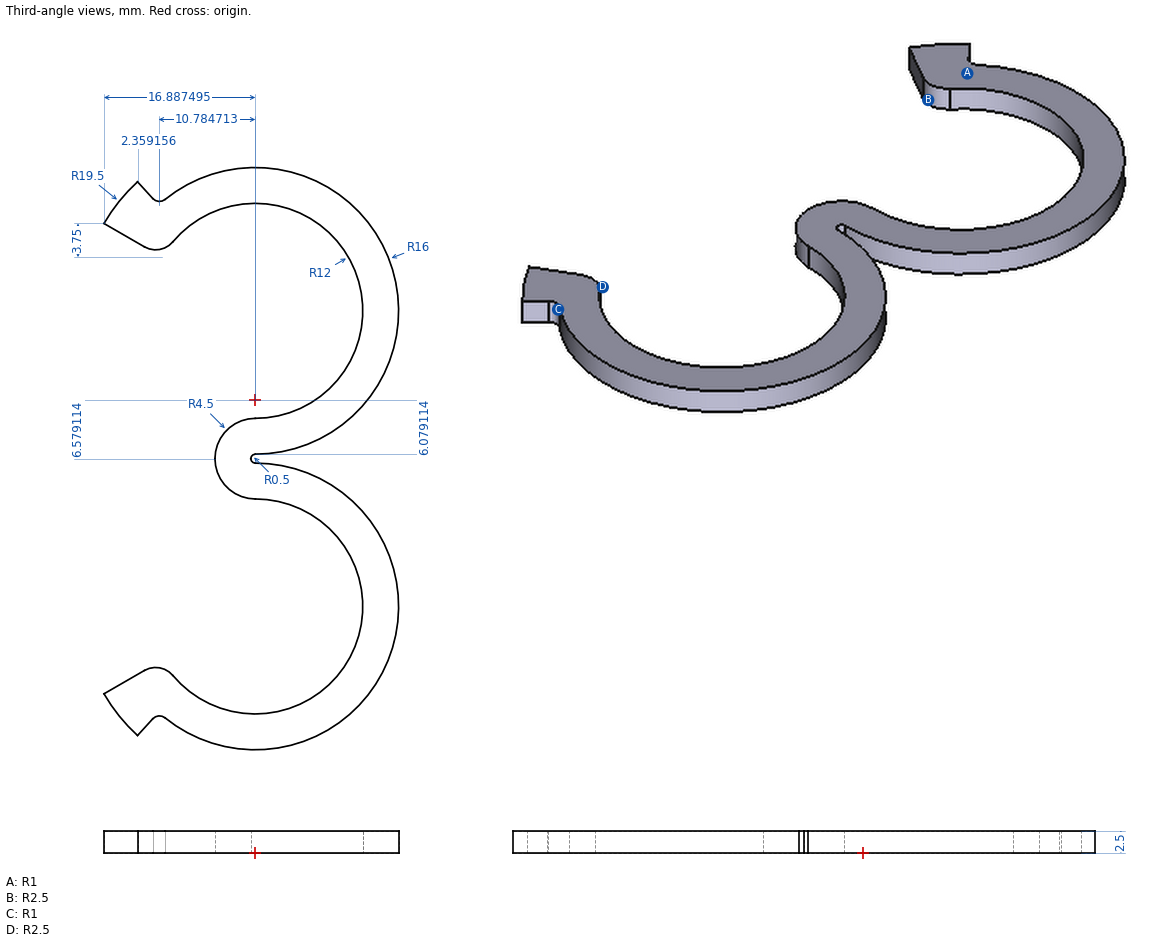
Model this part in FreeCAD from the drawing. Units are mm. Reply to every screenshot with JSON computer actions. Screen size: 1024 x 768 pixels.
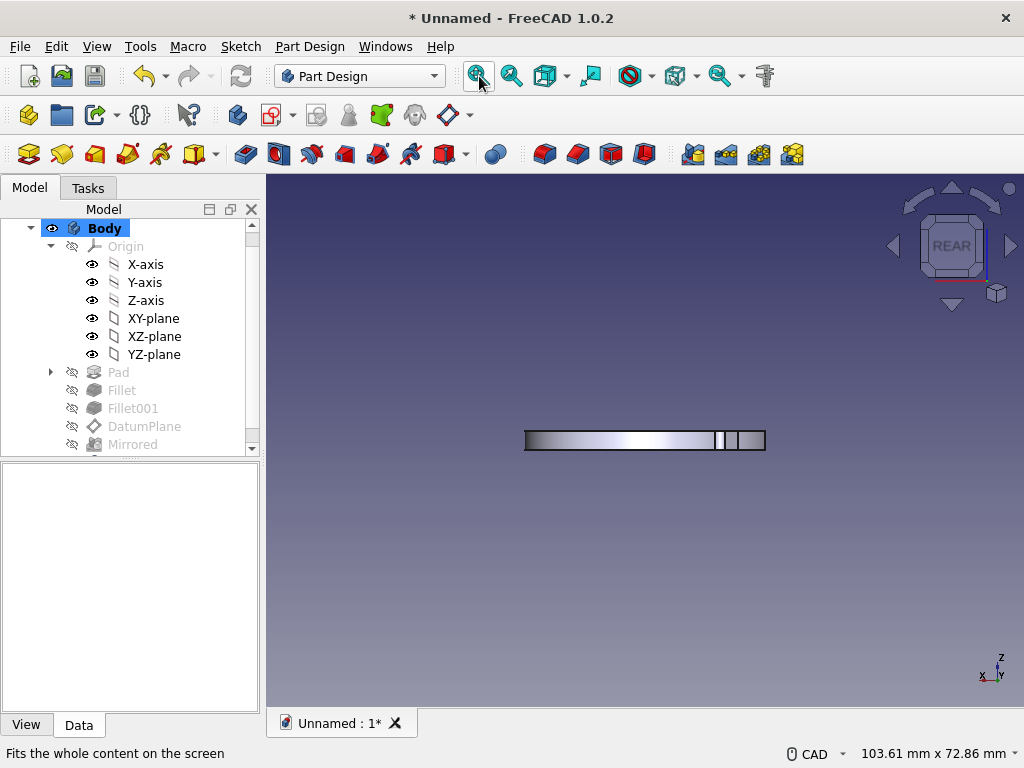
{"action": "key", "text": "6"}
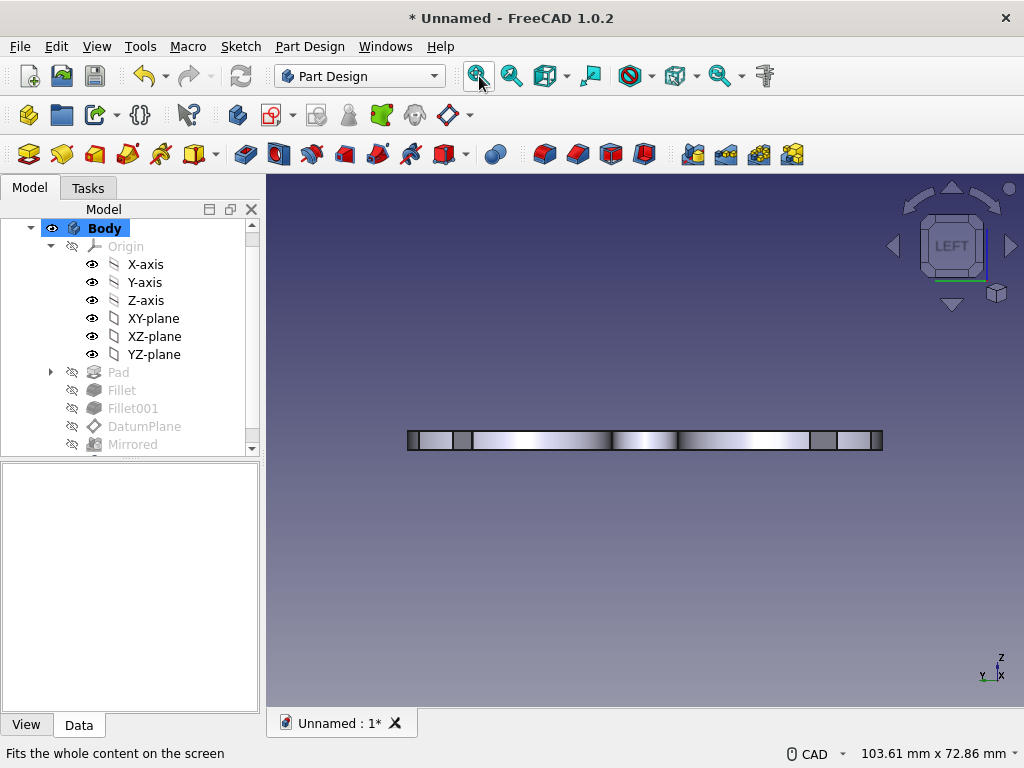
{"action": "scroll", "coordinate": [810, 439], "scroll_direction": "up", "scroll_amount": 4}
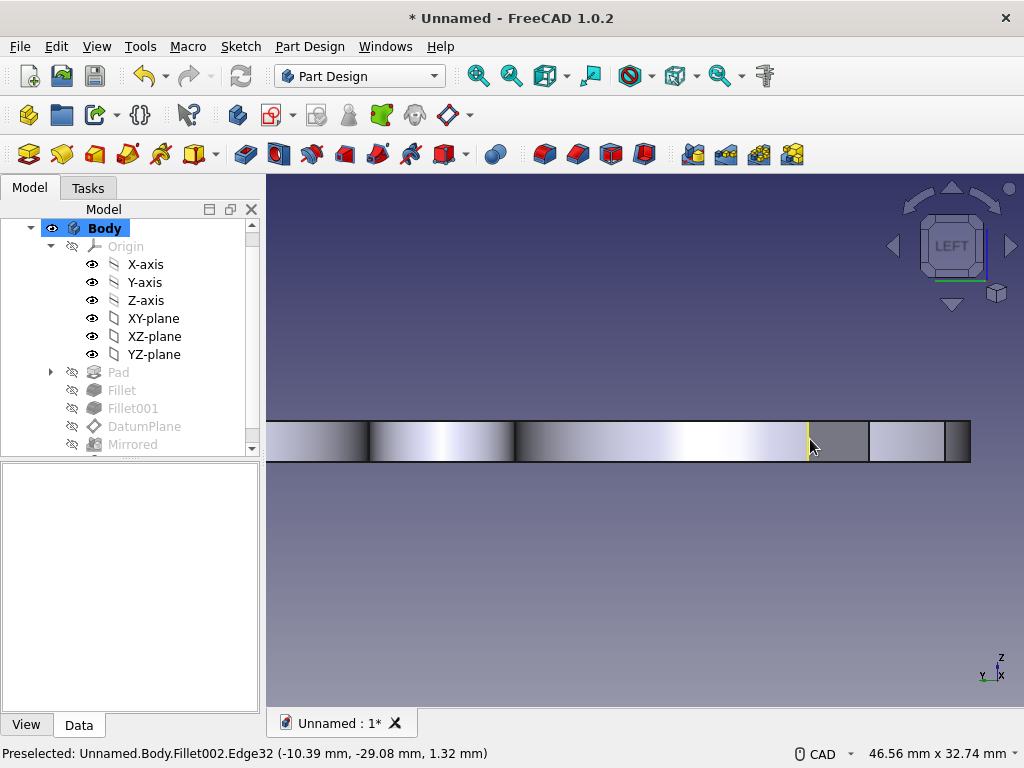
{"action": "left_click", "coordinate": [479, 76]}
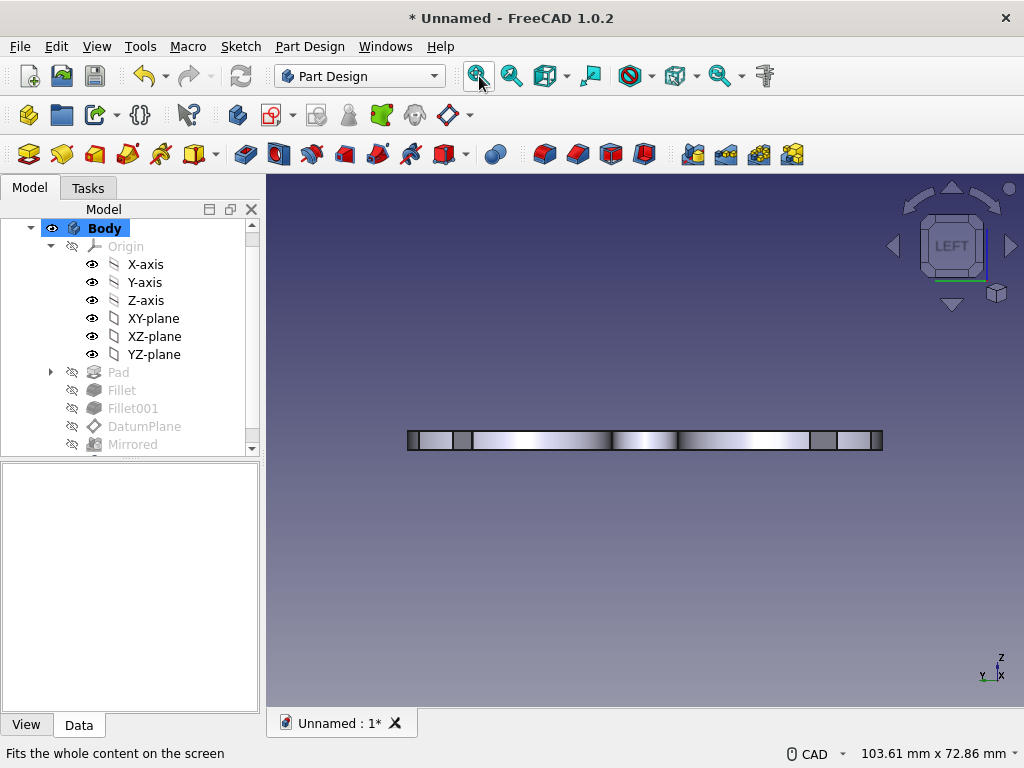
{"action": "key", "text": "v 3"}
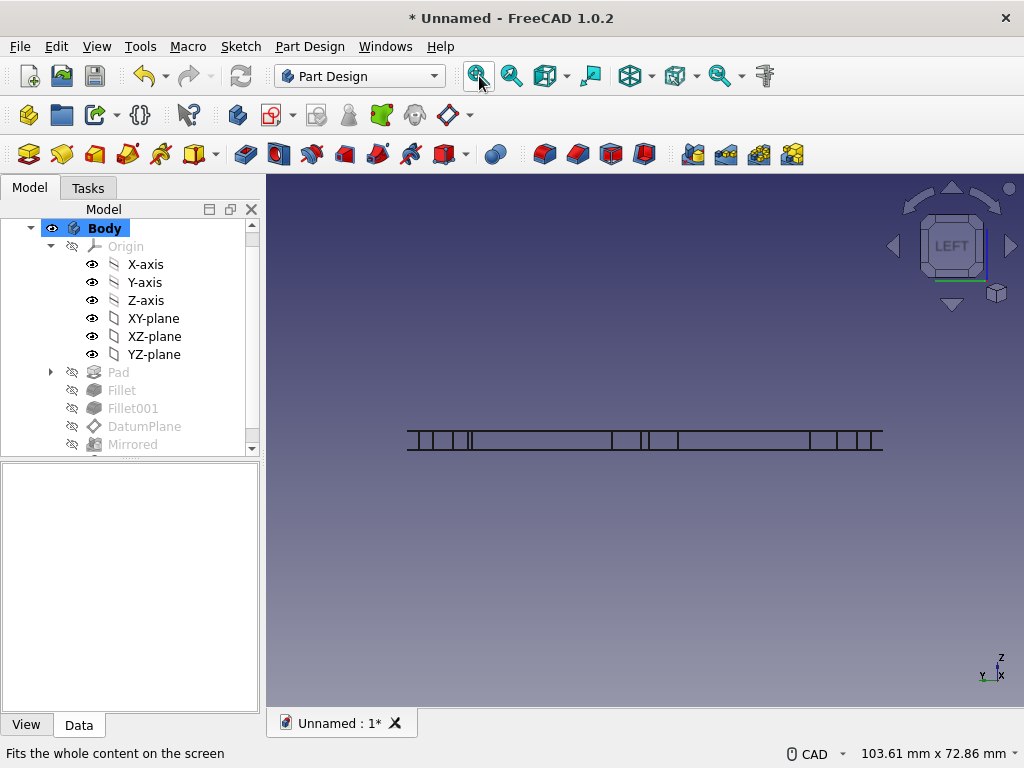
{"action": "key", "text": "0"}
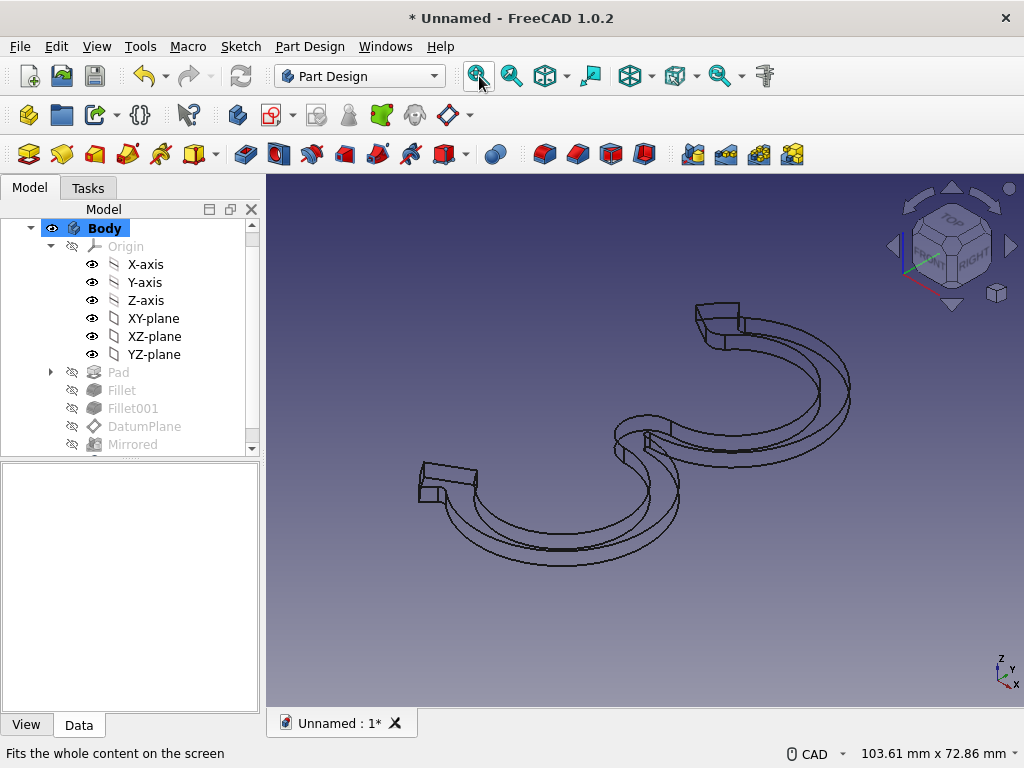
{"action": "scroll", "coordinate": [477, 477], "scroll_direction": "up", "scroll_amount": 4}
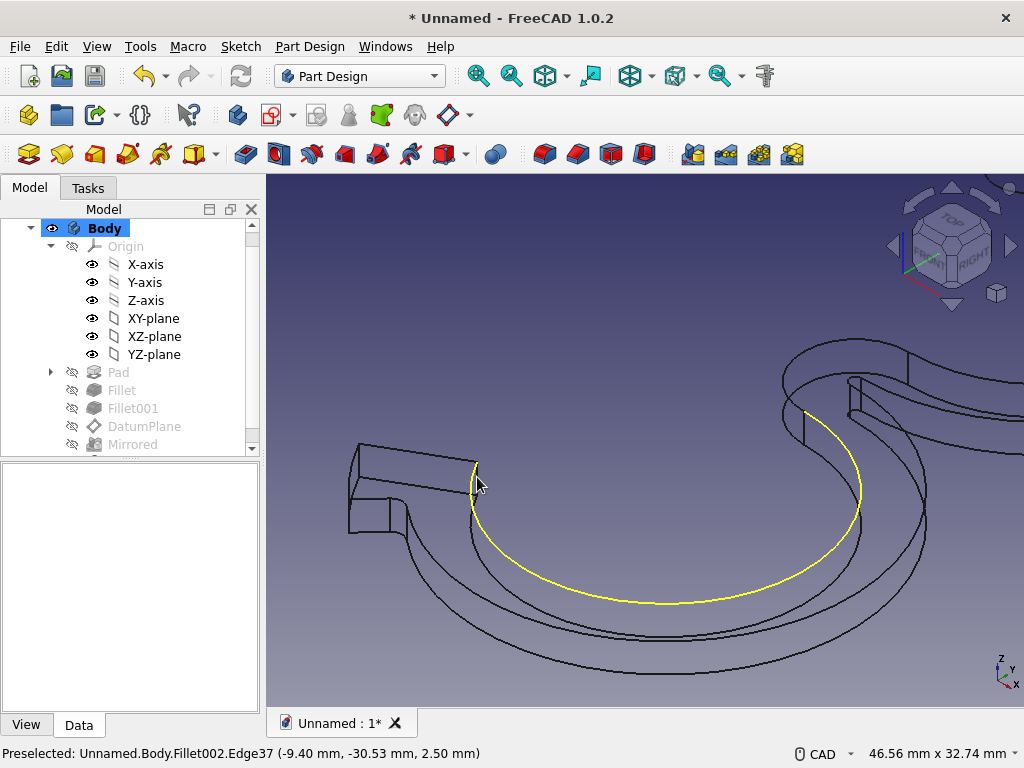
{"action": "left_click", "coordinate": [477, 488]}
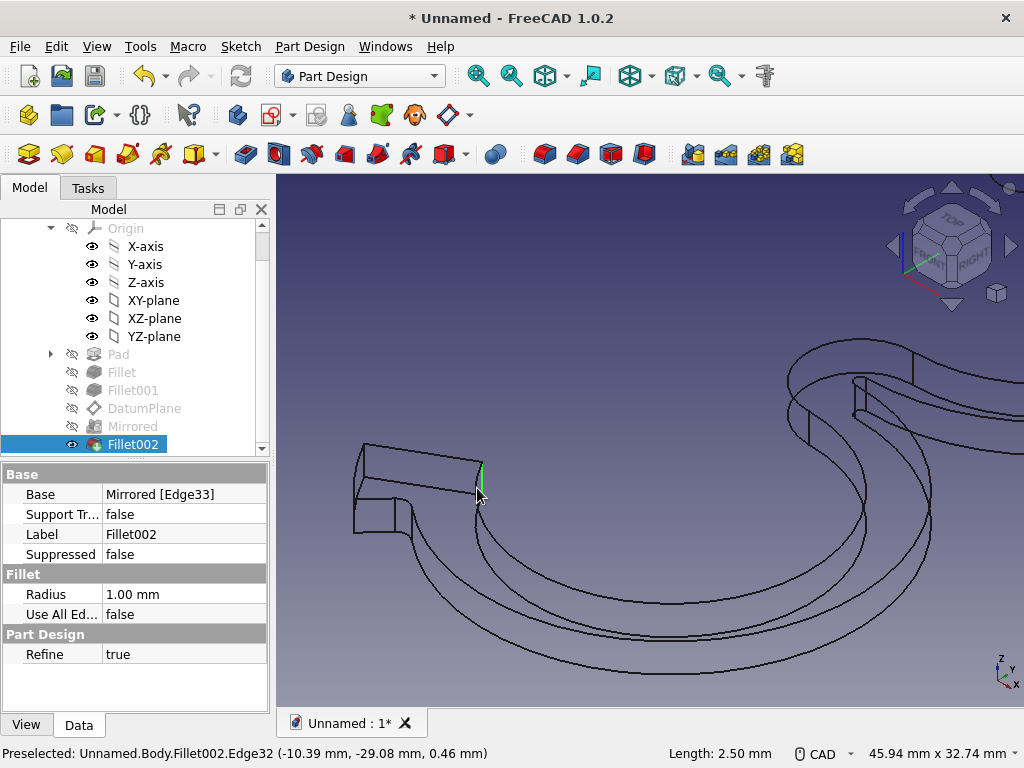
{"action": "key", "text": "v 1"}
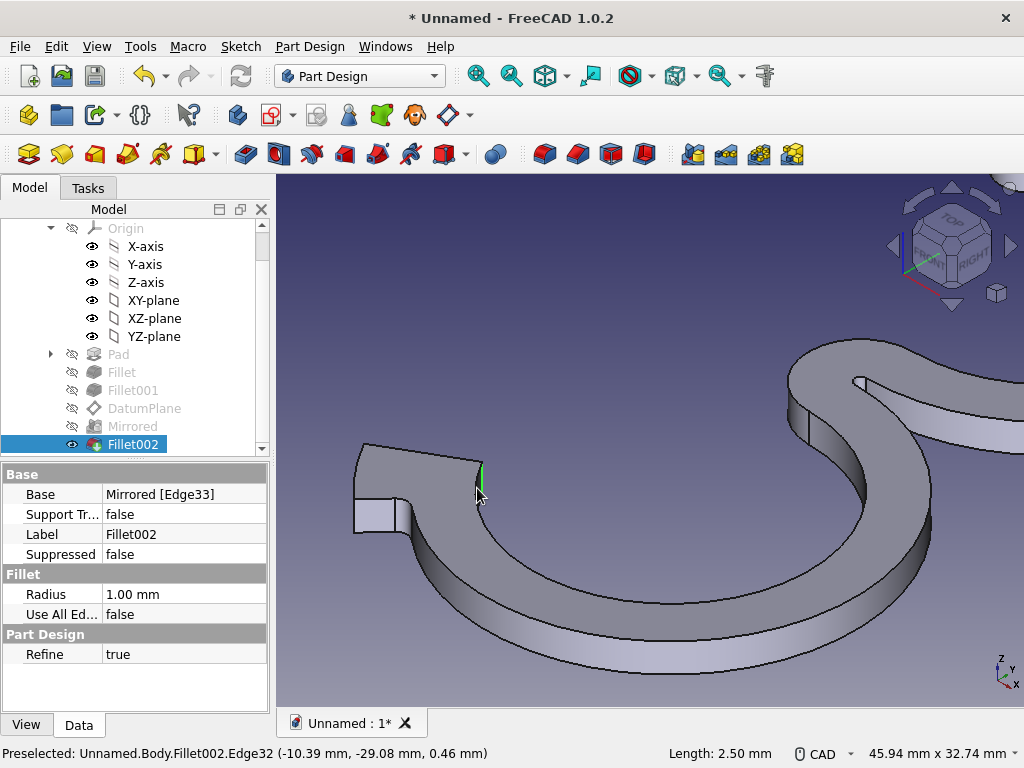
{"action": "left_click", "coordinate": [545, 154]}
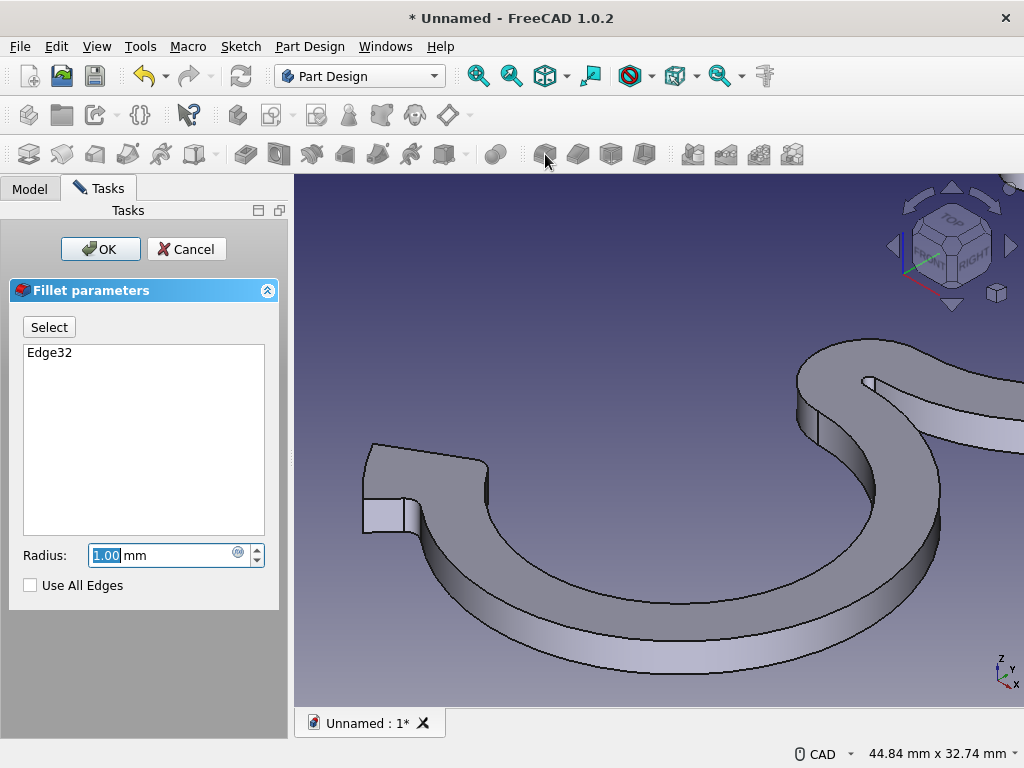
{"action": "type", "text": "2.5"}
{"action": "key", "text": "Tab"}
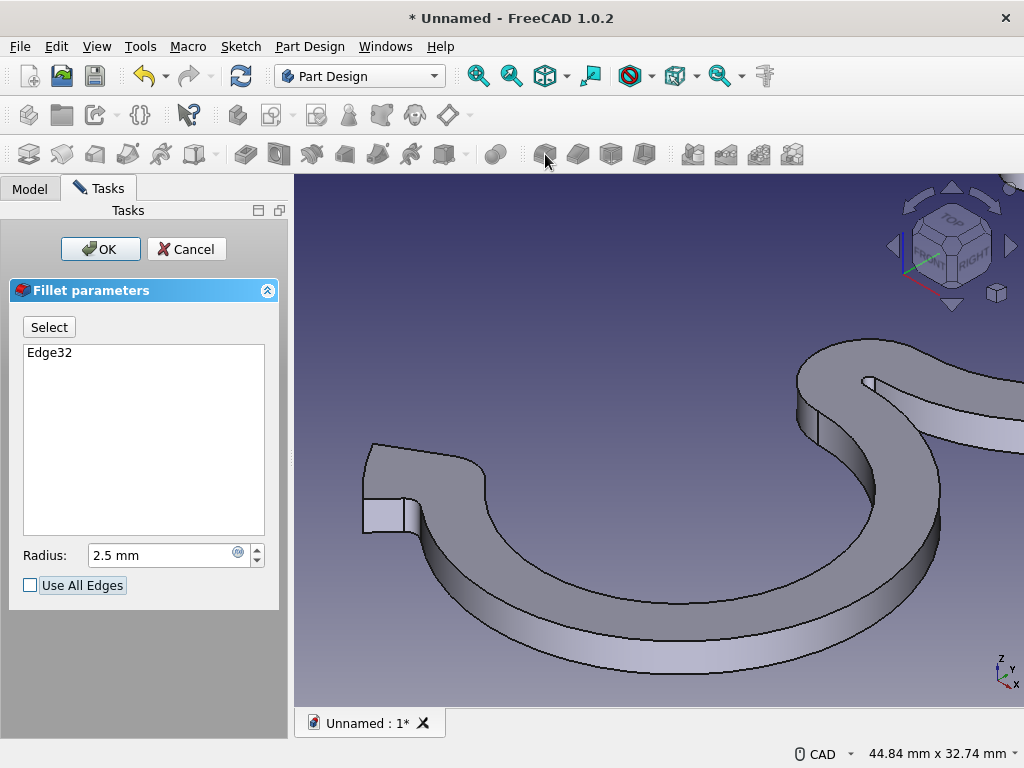
{"action": "left_click", "coordinate": [101, 249]}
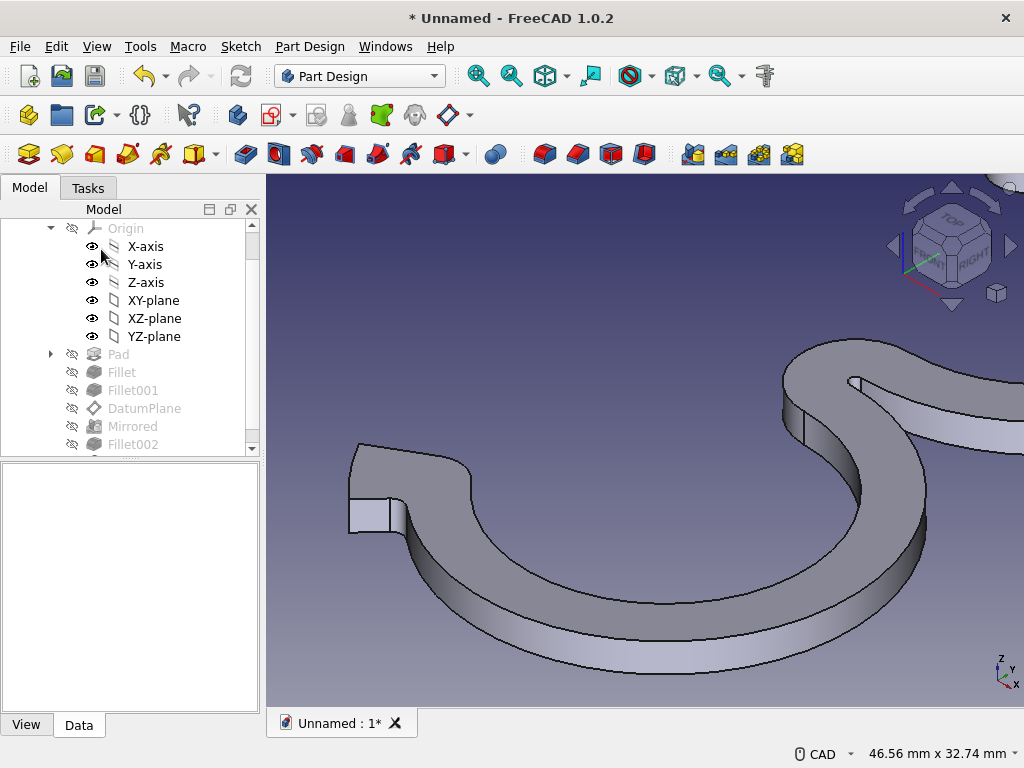
{"action": "left_click", "coordinate": [479, 76]}